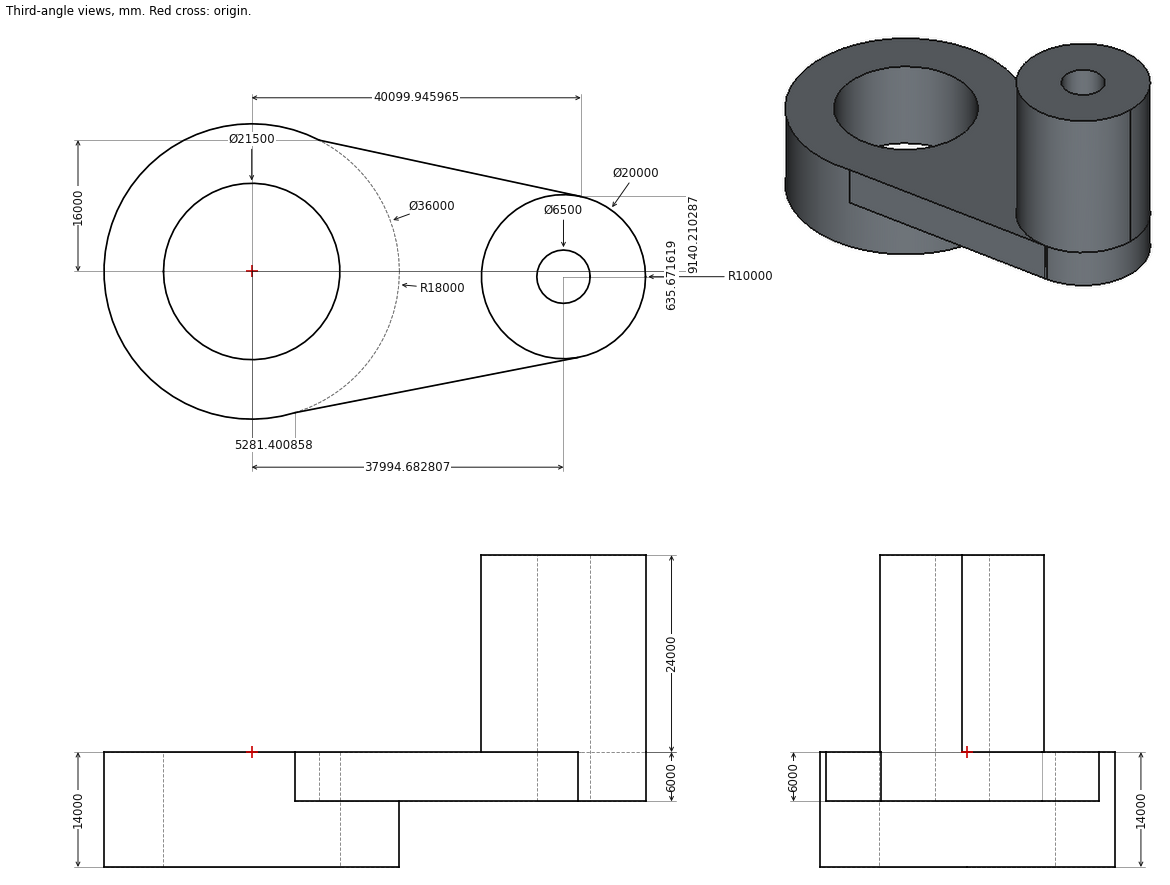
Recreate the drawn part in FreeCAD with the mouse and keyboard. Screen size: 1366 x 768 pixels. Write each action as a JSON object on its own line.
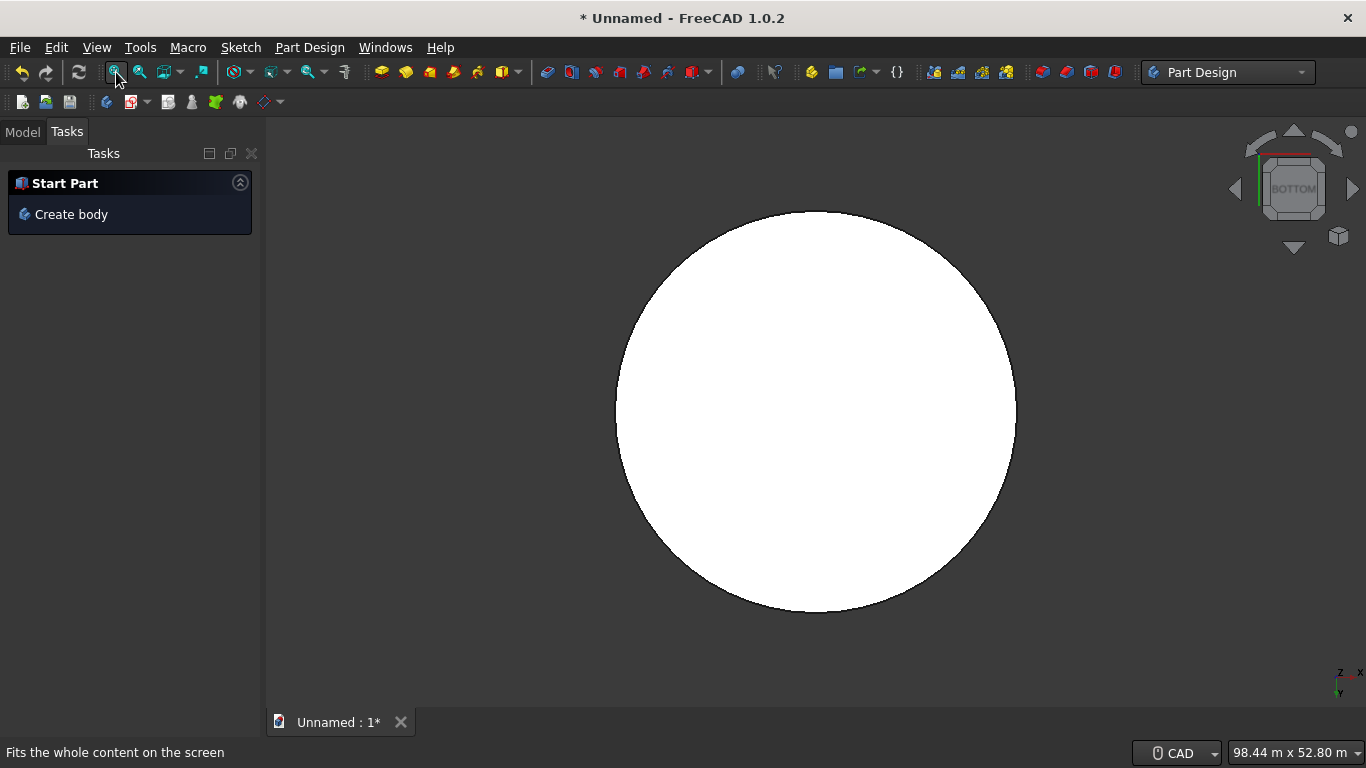
{"action": "left_click", "coordinate": [816, 411]}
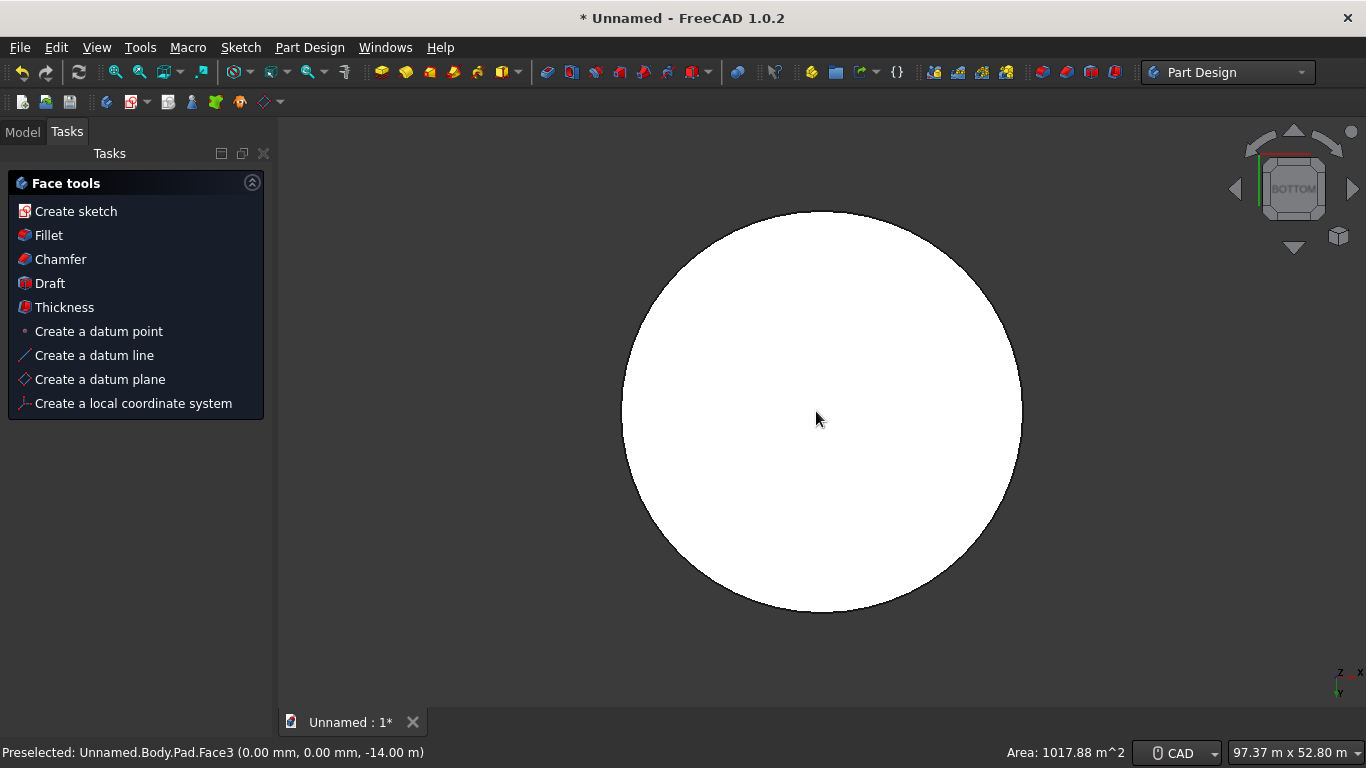
{"action": "left_click", "coordinate": [132, 102]}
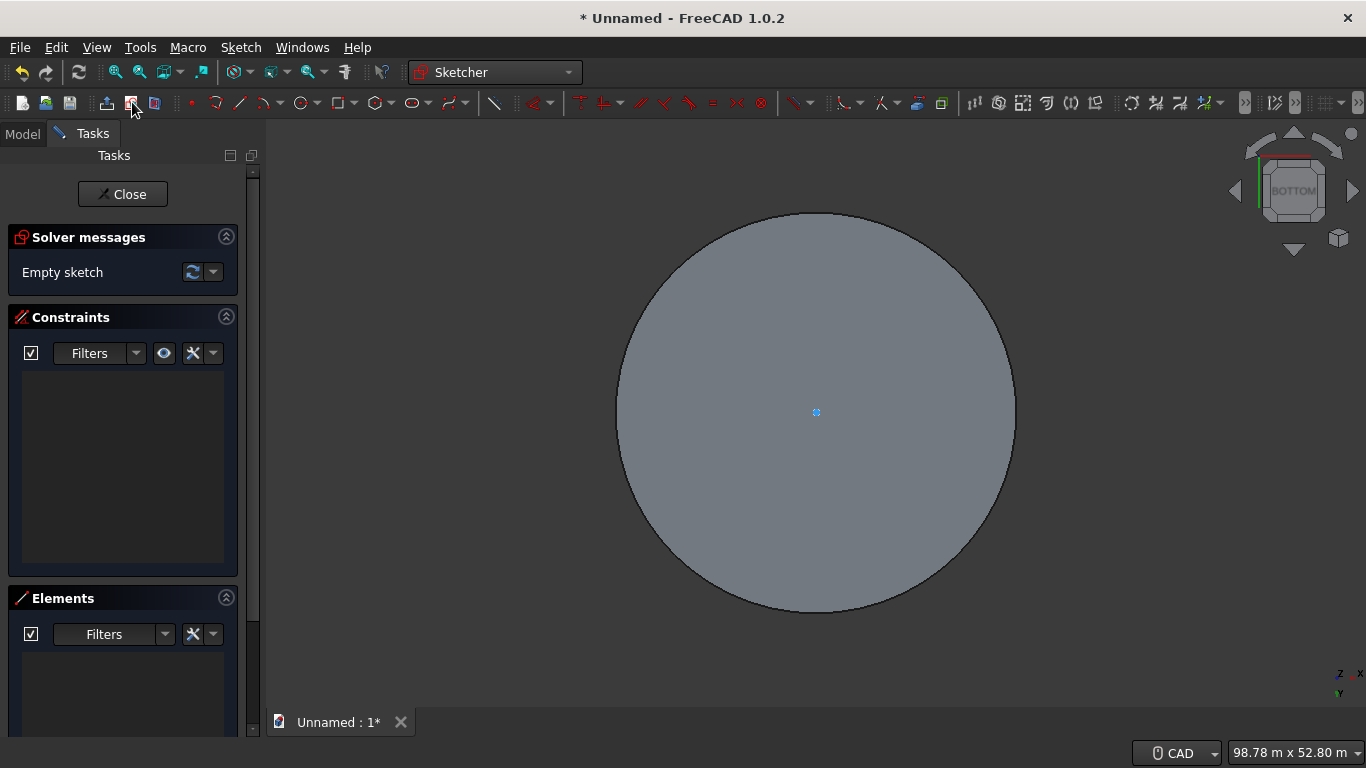
{"action": "scroll", "coordinate": [955, 413], "scroll_direction": "up", "scroll_amount": 2}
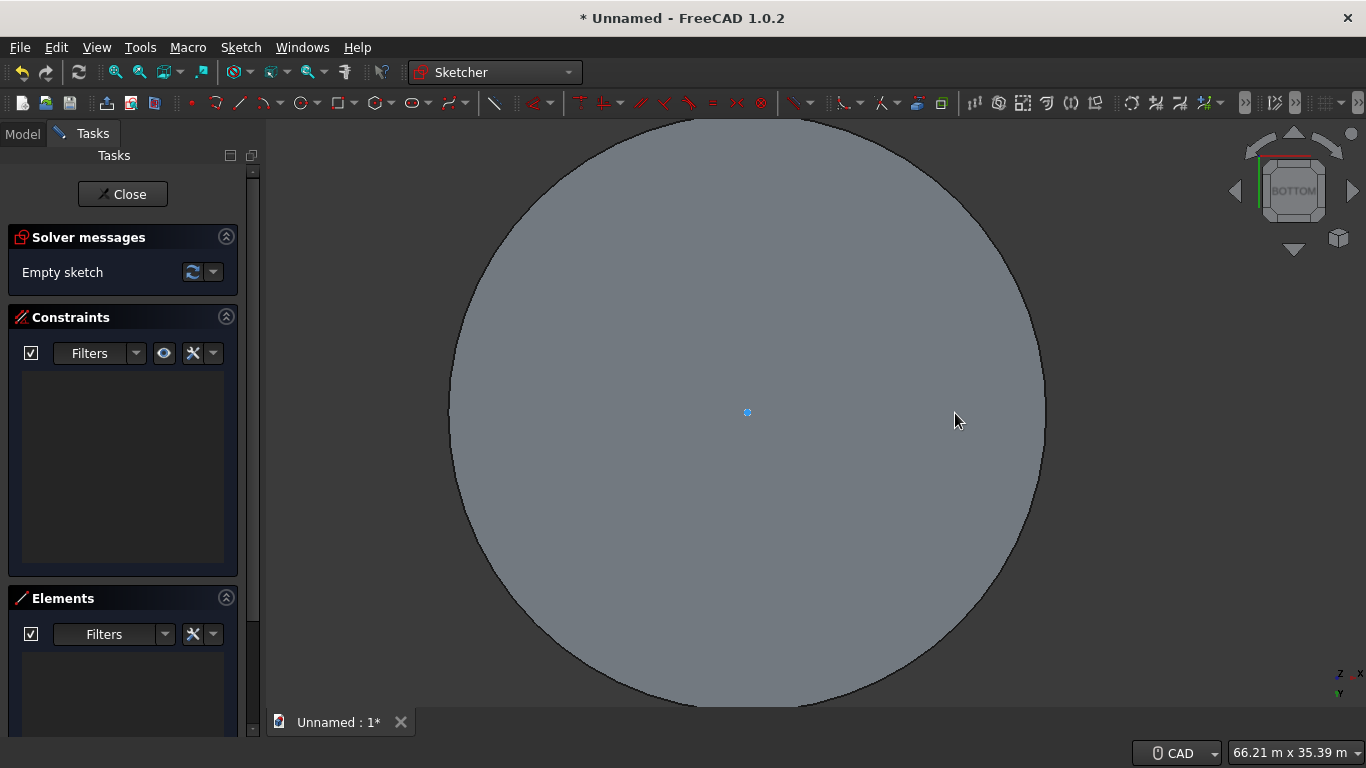
{"action": "left_click", "coordinate": [302, 104]}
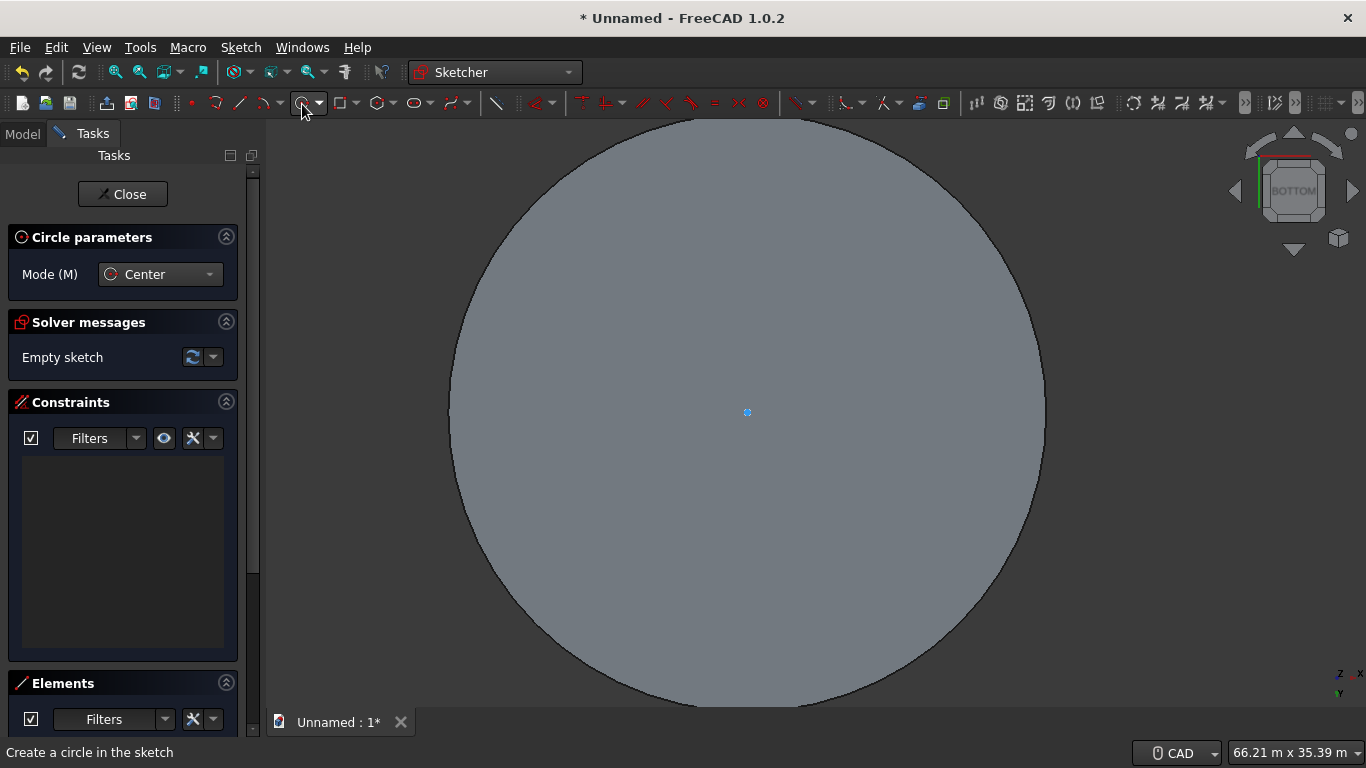
{"action": "left_click", "coordinate": [747, 413]}
{"action": "left_click", "coordinate": [874, 286]}
{"action": "key", "text": "Escape"}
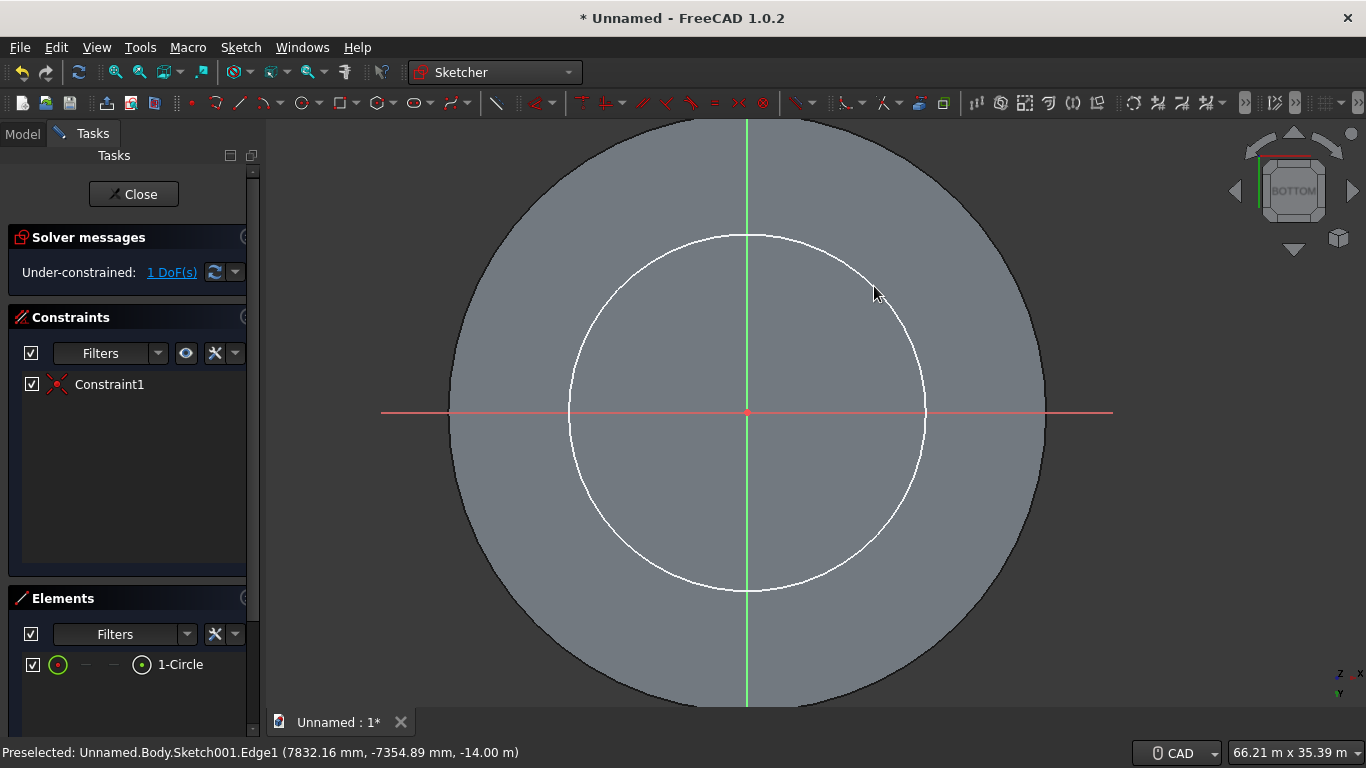
{"action": "left_click", "coordinate": [536, 104]}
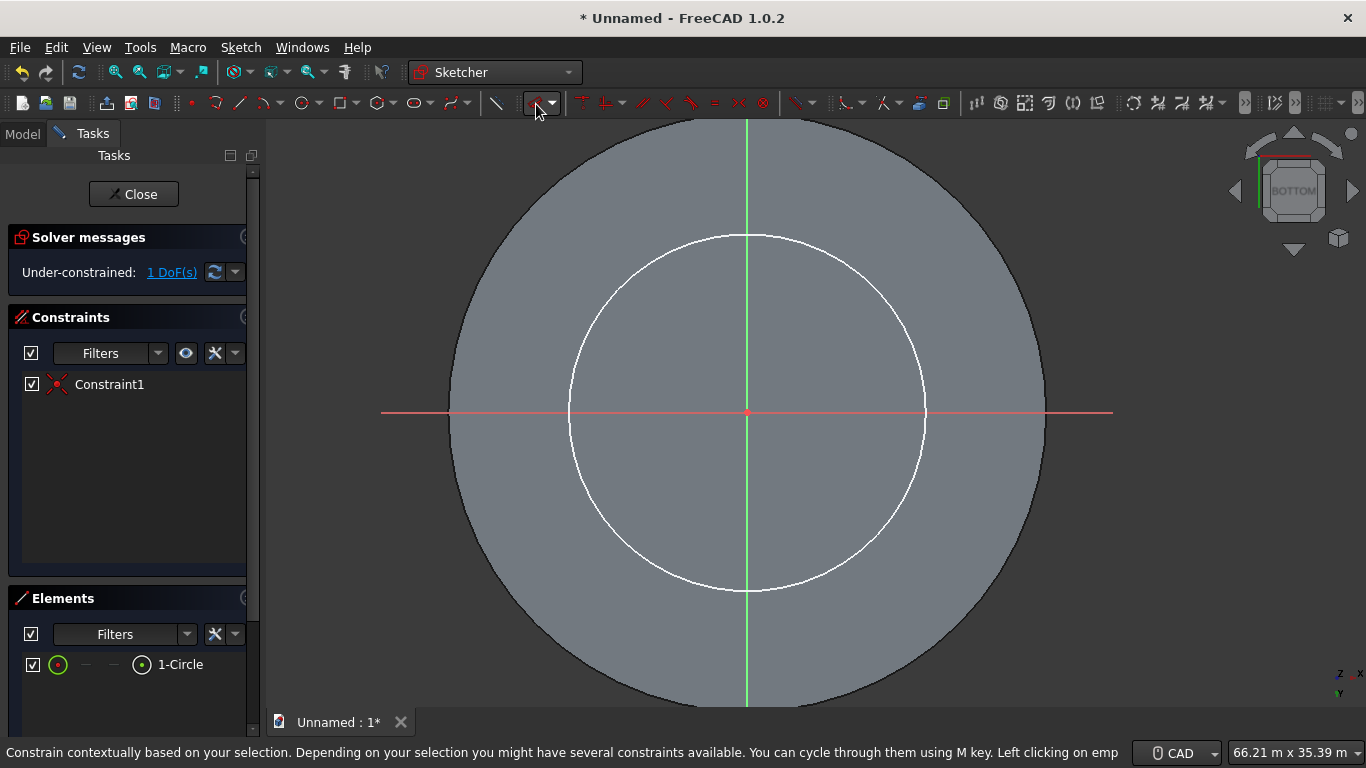
{"action": "left_click", "coordinate": [873, 286]}
{"action": "left_click", "coordinate": [896, 263]}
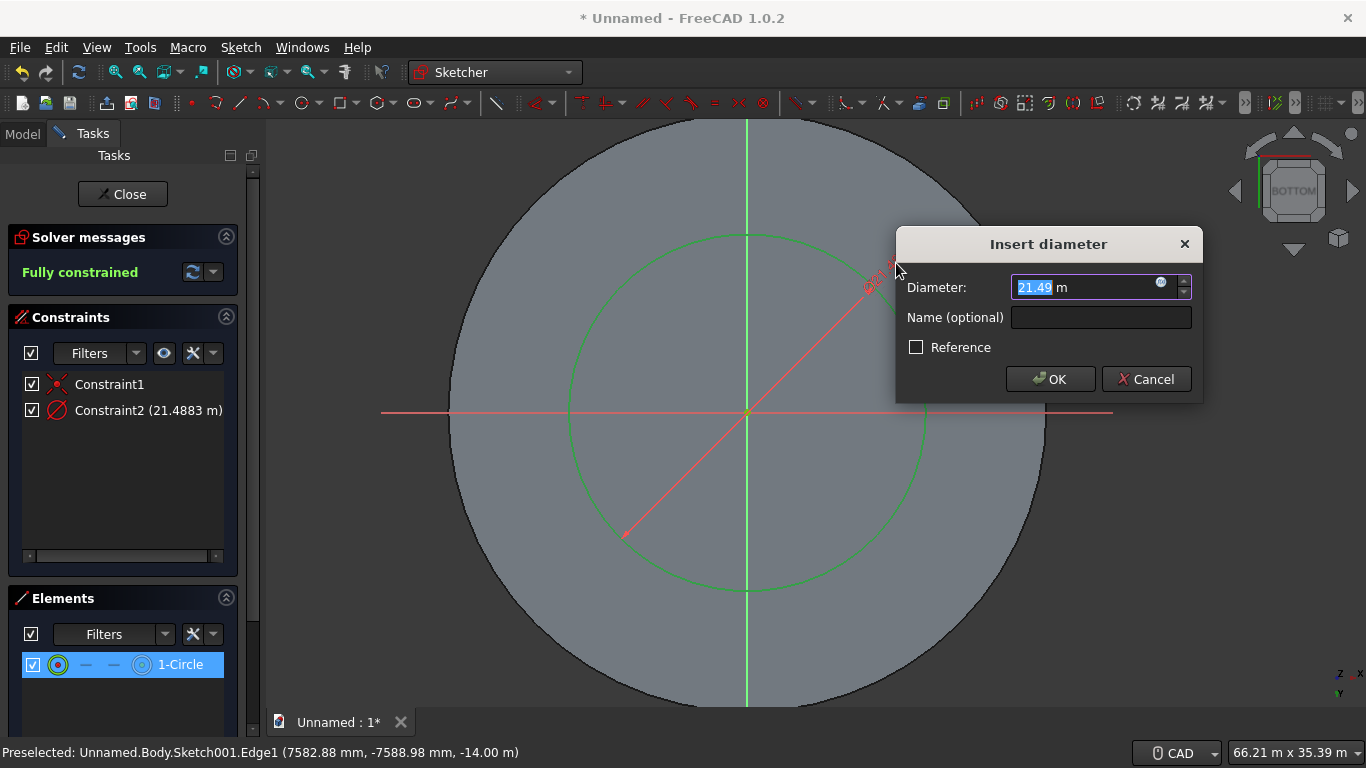
{"action": "key", "text": "ctrl+a"}
{"action": "type", "text": "21500 mm"}
{"action": "key", "text": "Return"}
{"action": "key", "text": "Escape"}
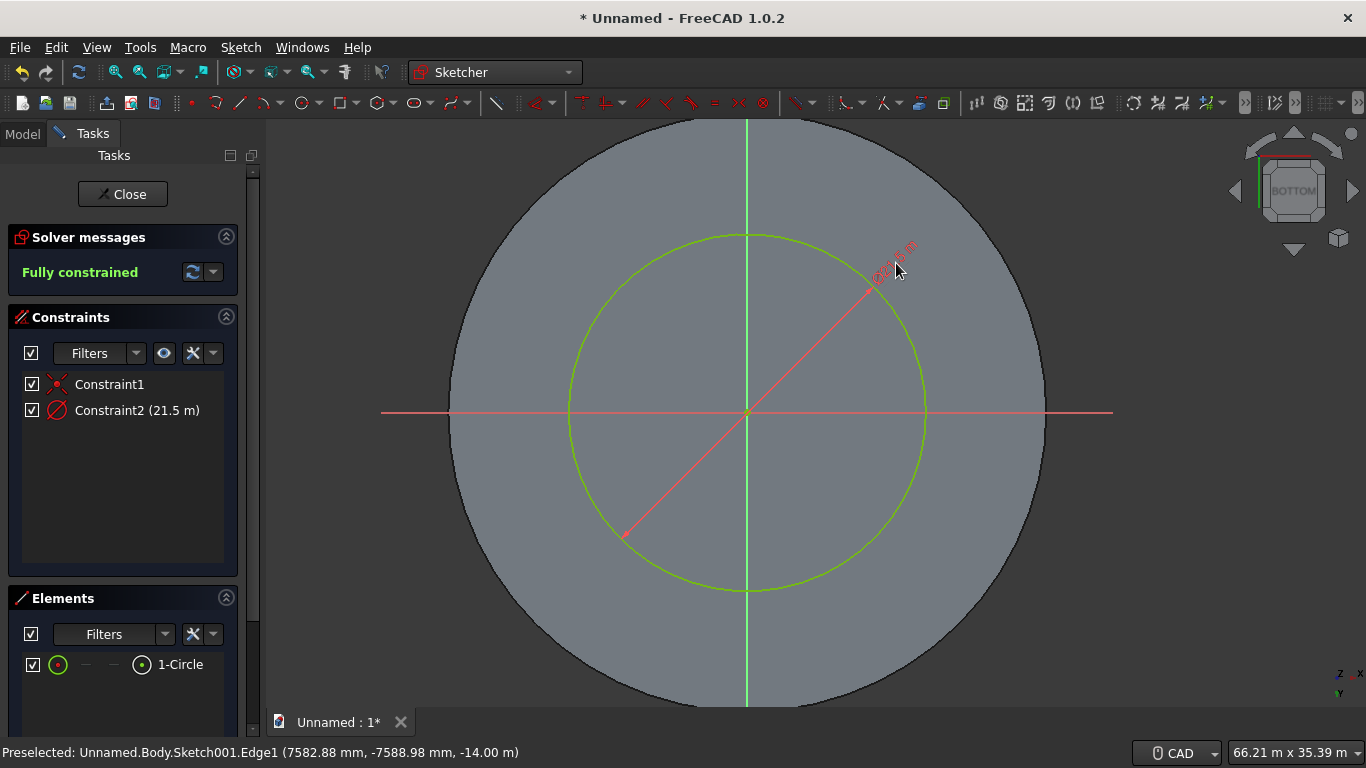
{"action": "left_click", "coordinate": [123, 194]}